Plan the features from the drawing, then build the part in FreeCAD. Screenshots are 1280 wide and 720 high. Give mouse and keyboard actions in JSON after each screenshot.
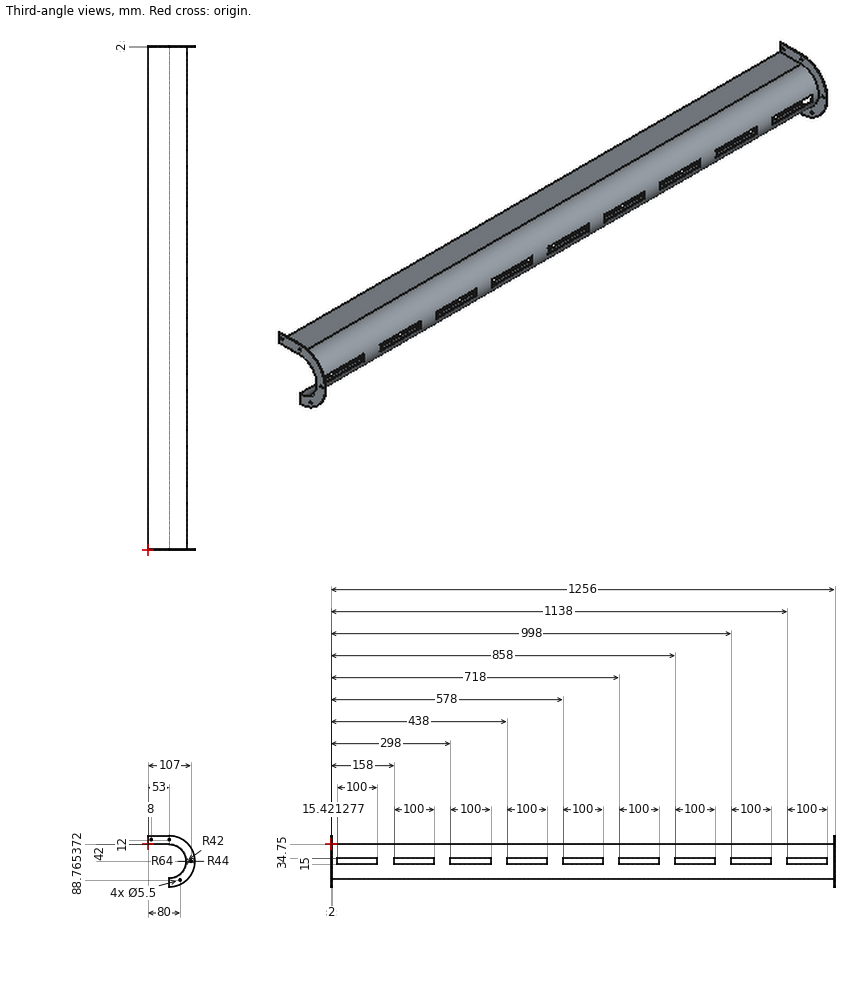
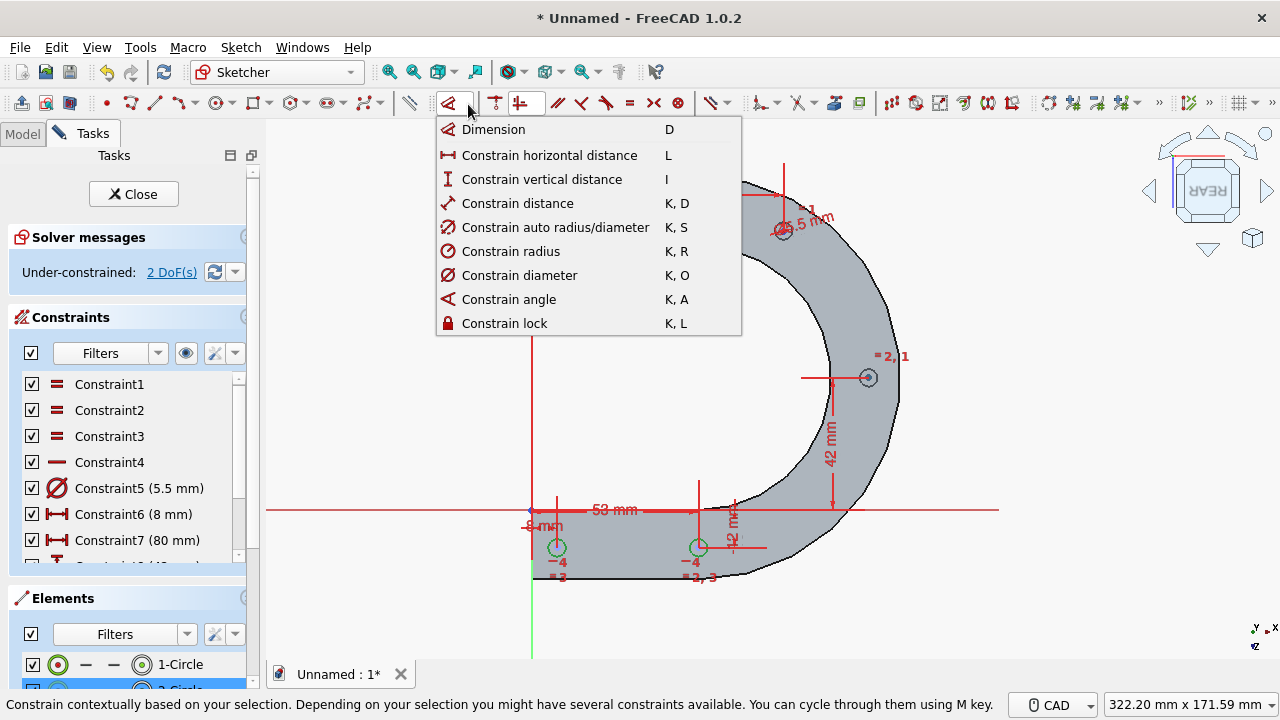
{"action": "left_click", "coordinate": [589, 155]}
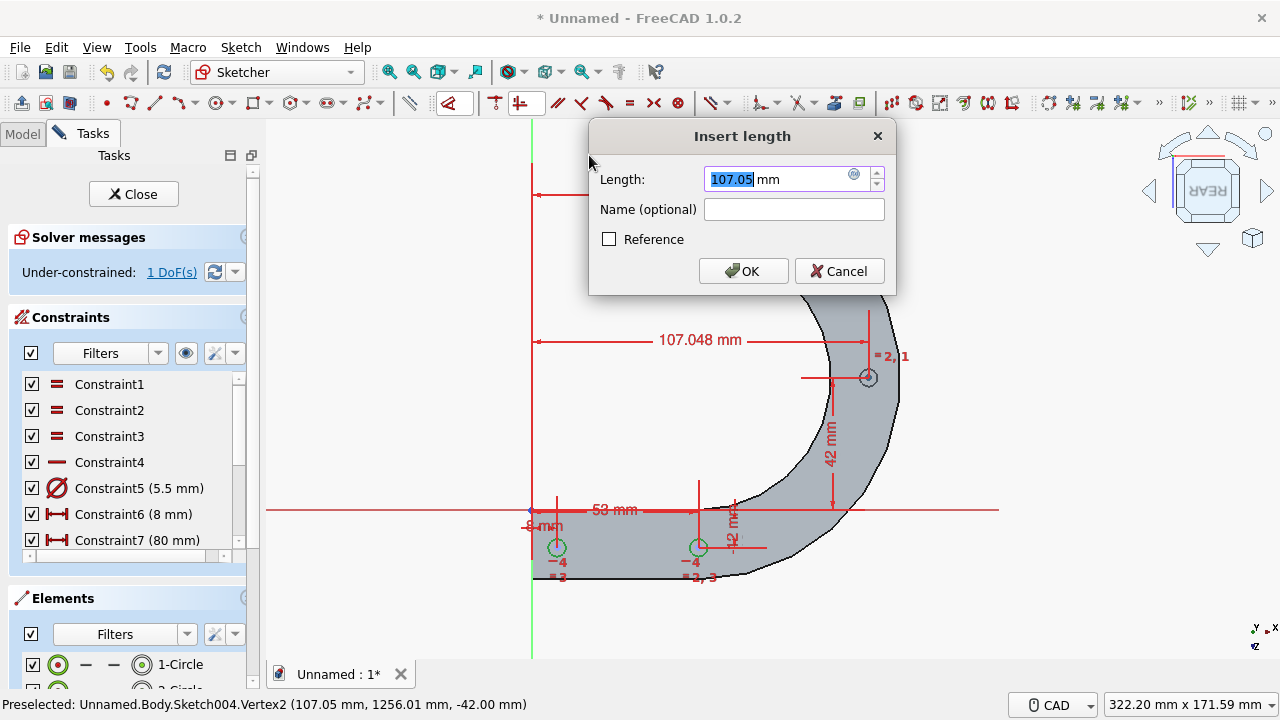
{"action": "type", "text": "107"}
{"action": "key", "text": "Return"}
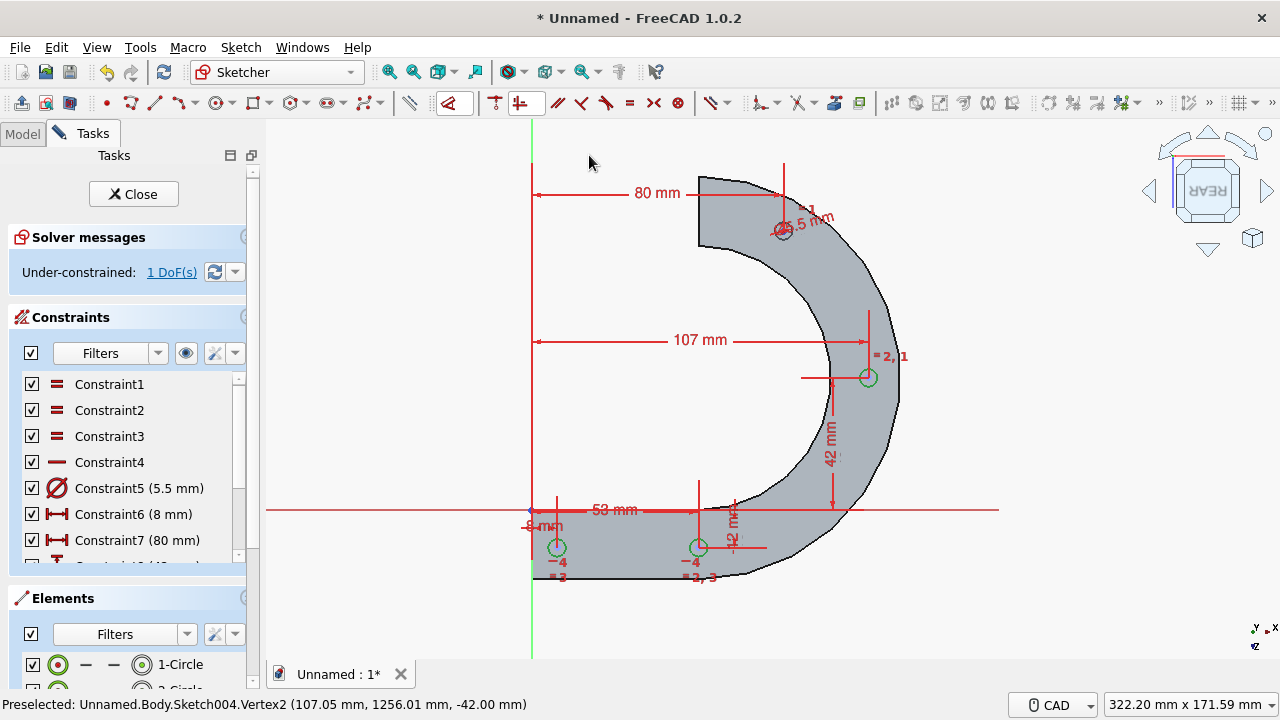
{"action": "left_click", "coordinate": [784, 231]}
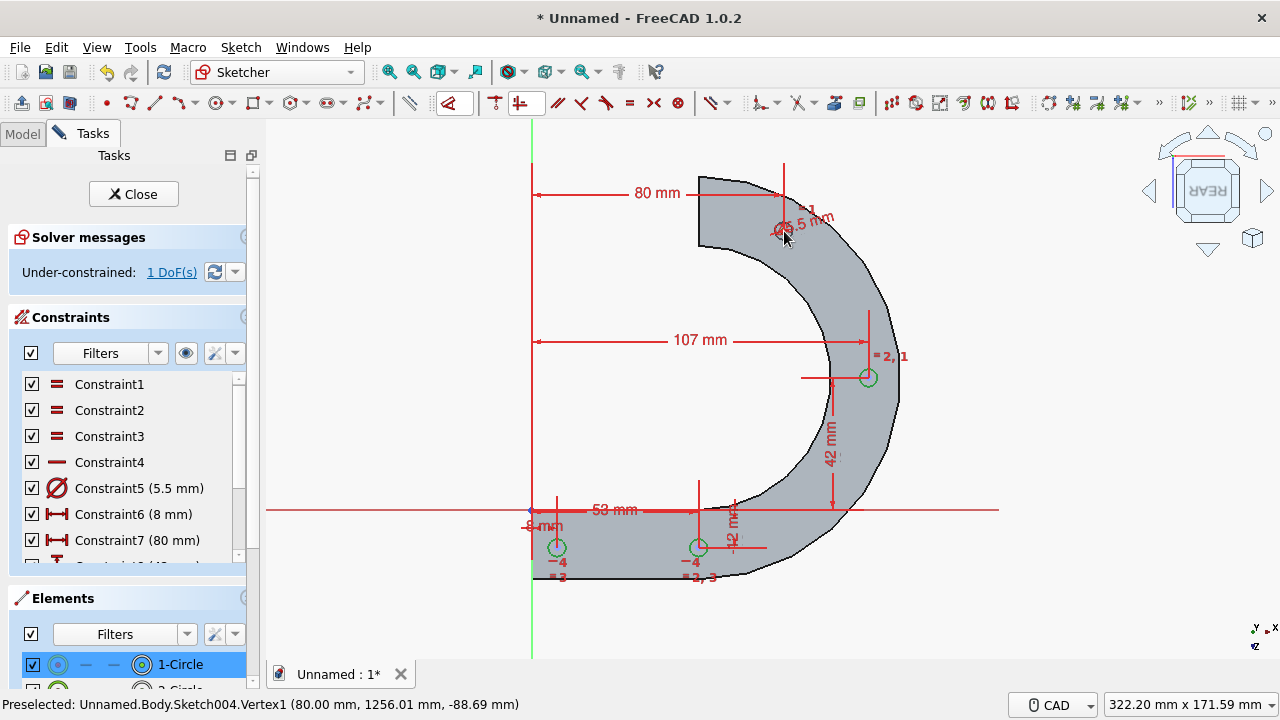
{"action": "key", "text": "i"}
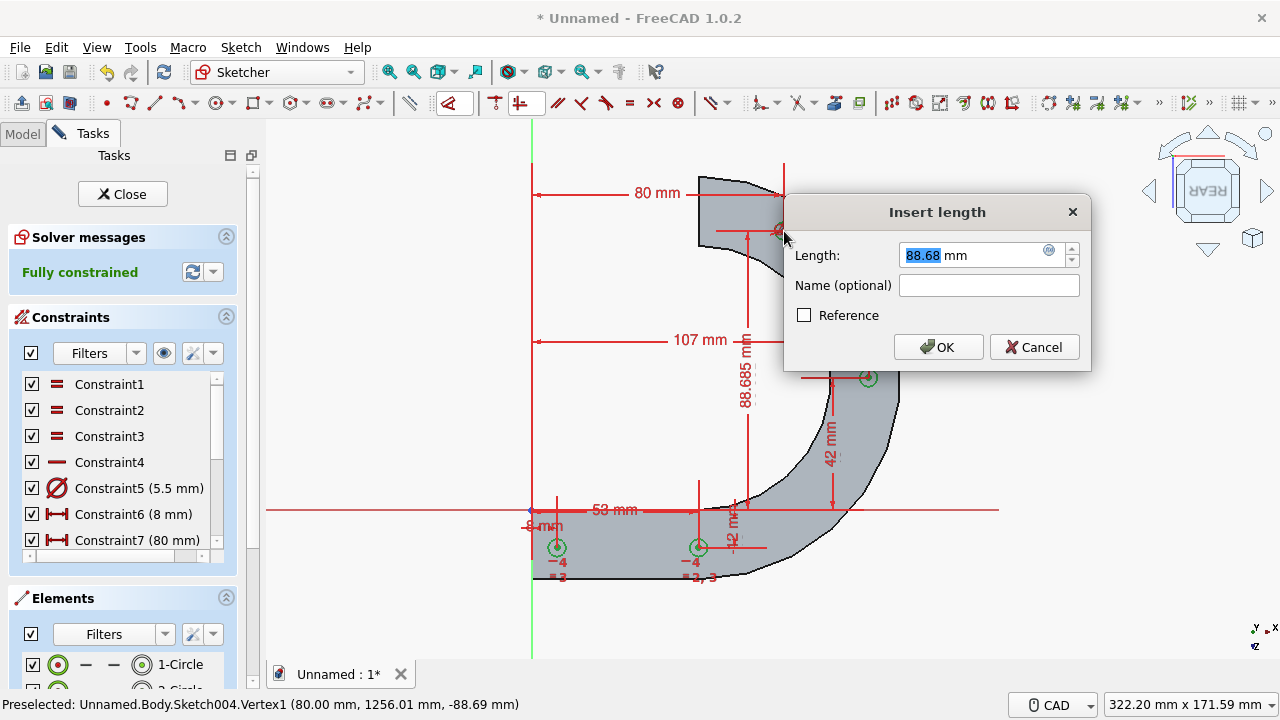
{"action": "type", "text": "88.765372"}
{"action": "key", "text": "Return"}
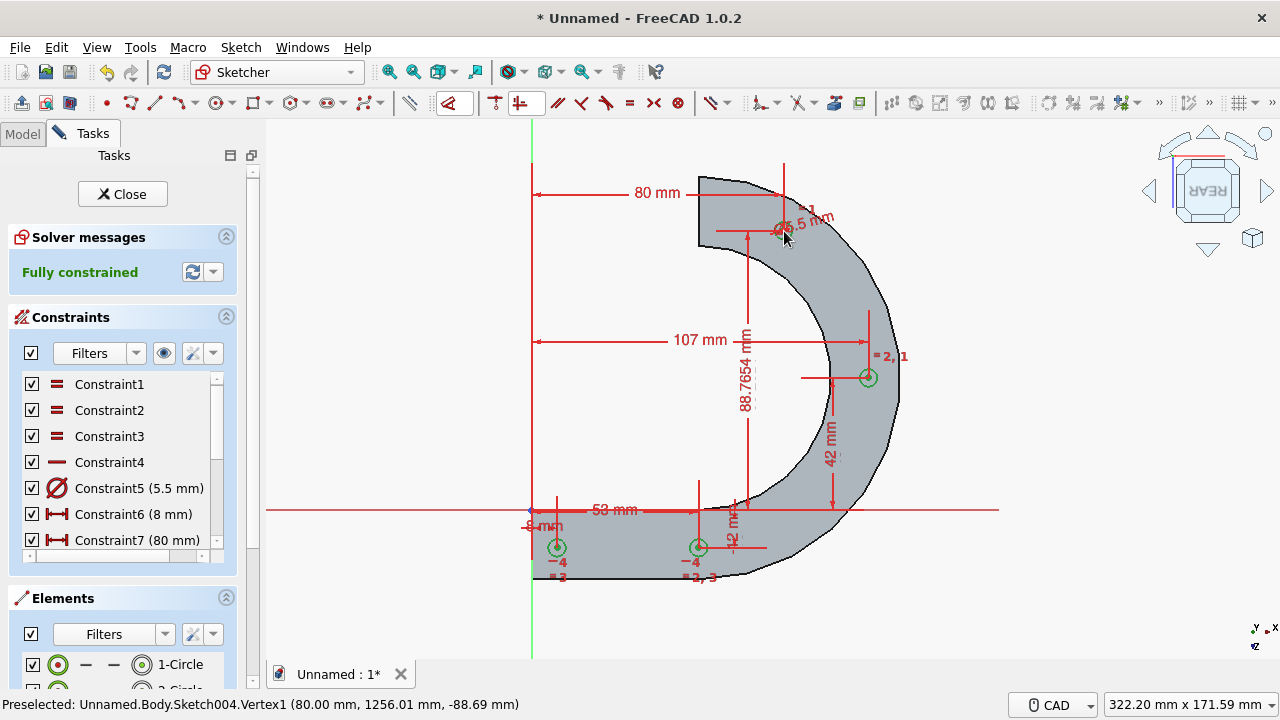
{"action": "left_click", "coordinate": [123, 194]}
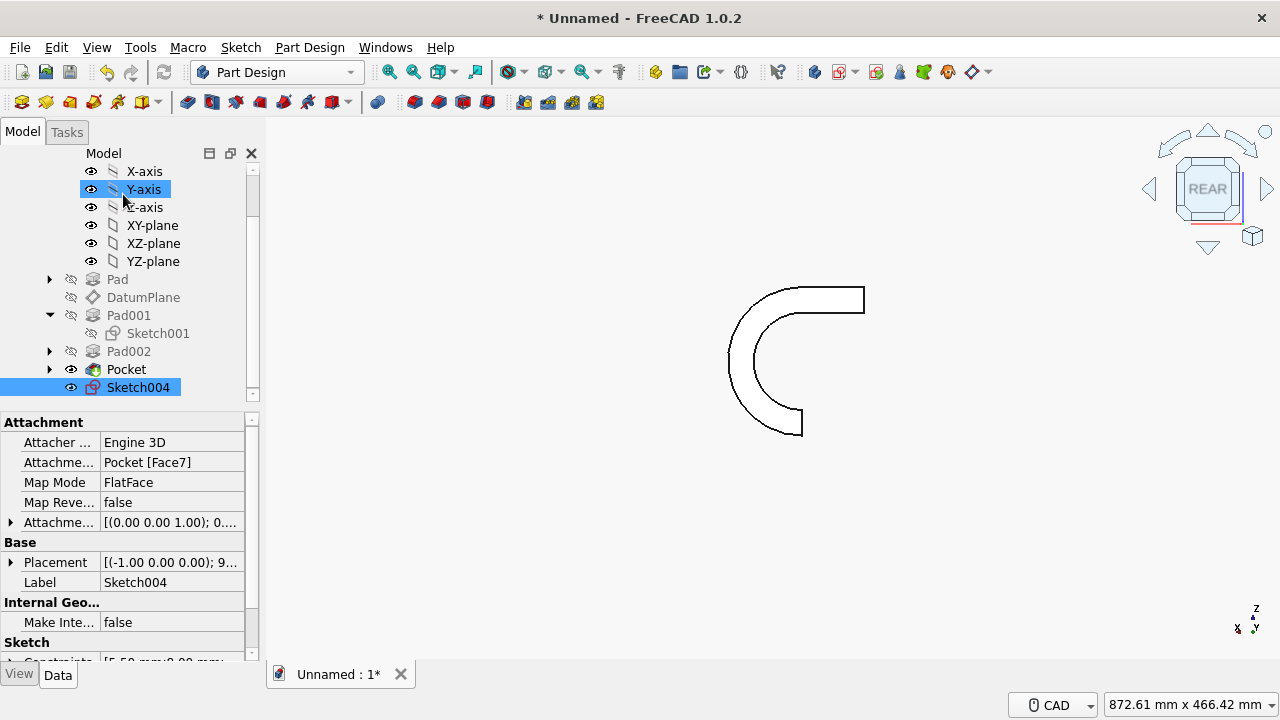
{"action": "left_click", "coordinate": [188, 102]}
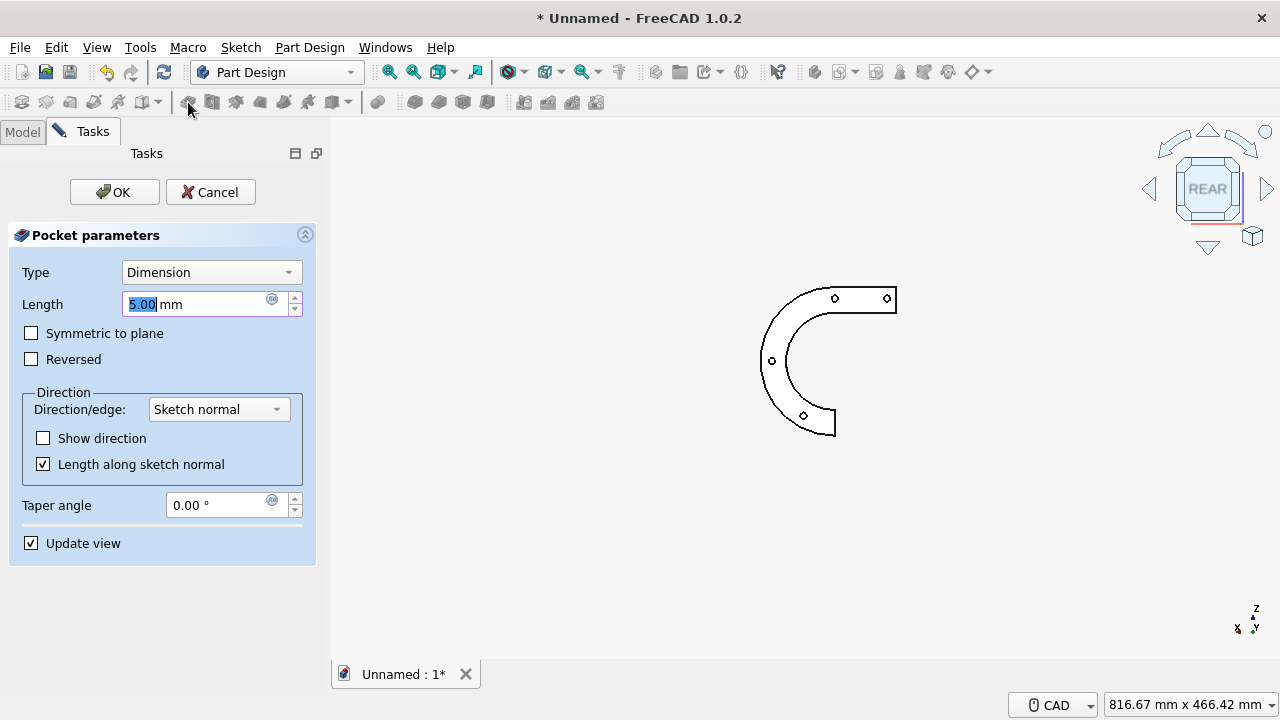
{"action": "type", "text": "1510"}
{"action": "key", "text": "Tab"}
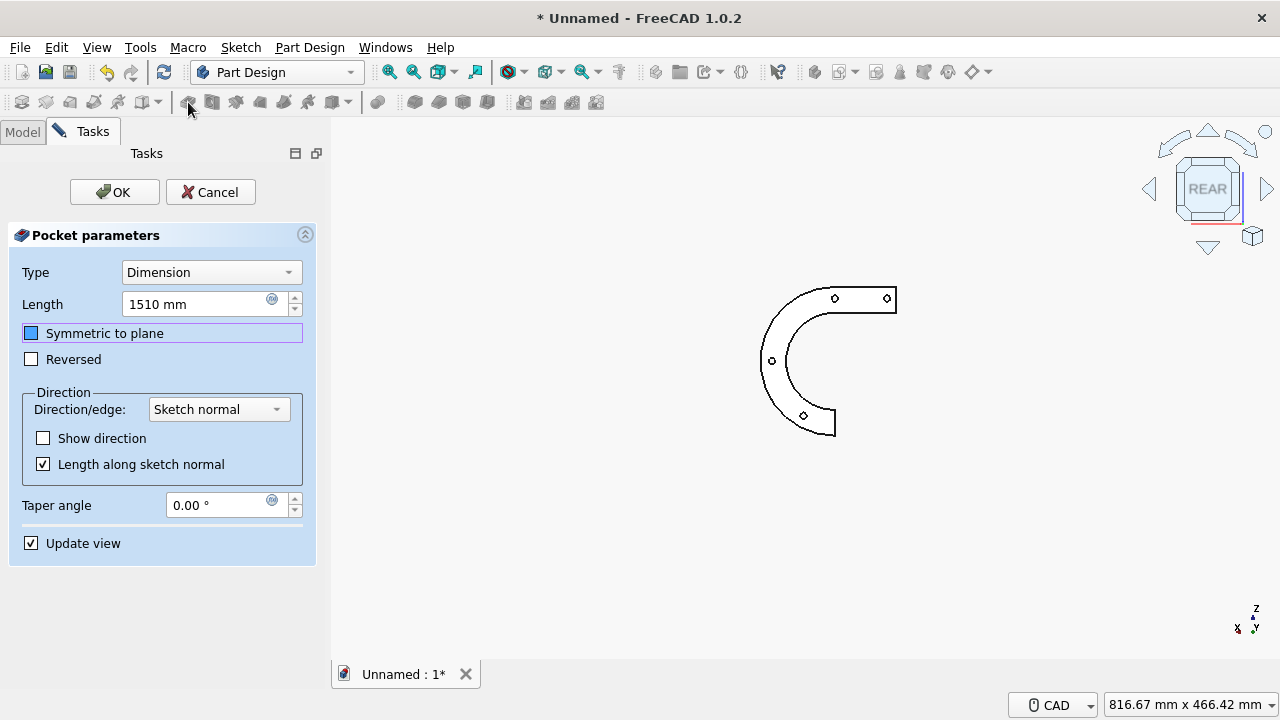
{"action": "left_click", "coordinate": [115, 192]}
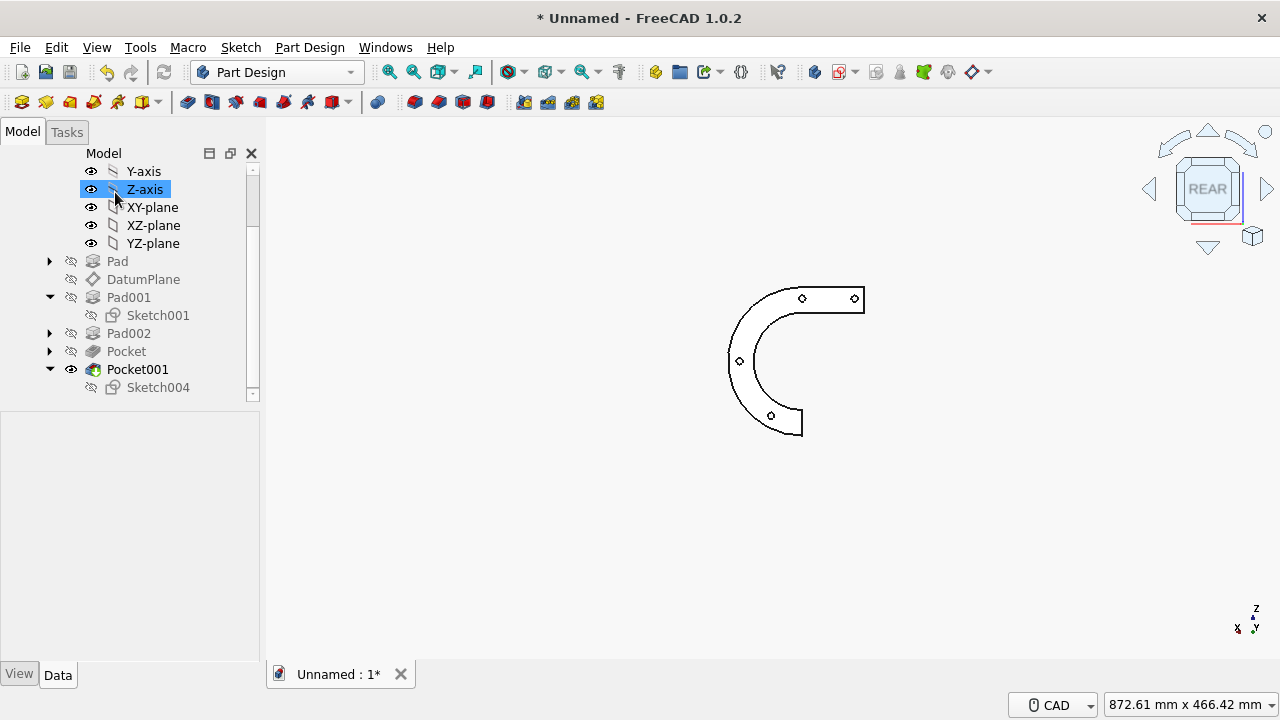
{"action": "key", "text": "0"}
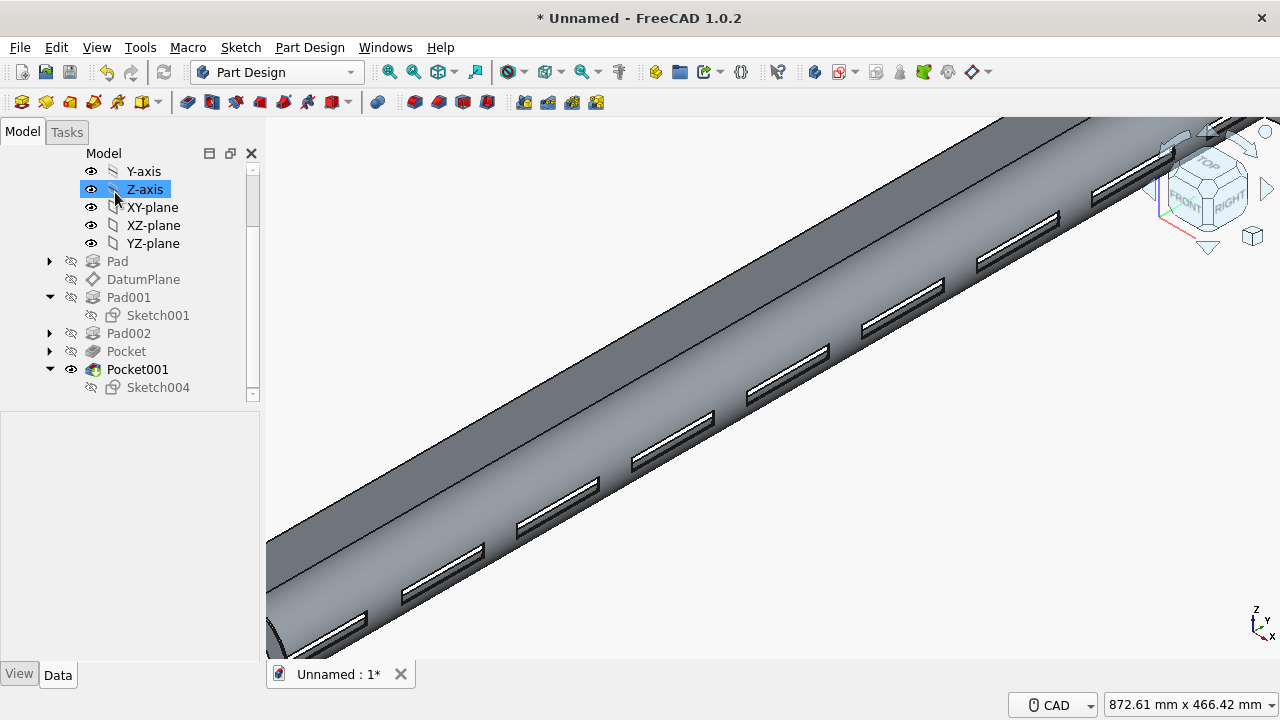
{"action": "left_click", "coordinate": [390, 72]}